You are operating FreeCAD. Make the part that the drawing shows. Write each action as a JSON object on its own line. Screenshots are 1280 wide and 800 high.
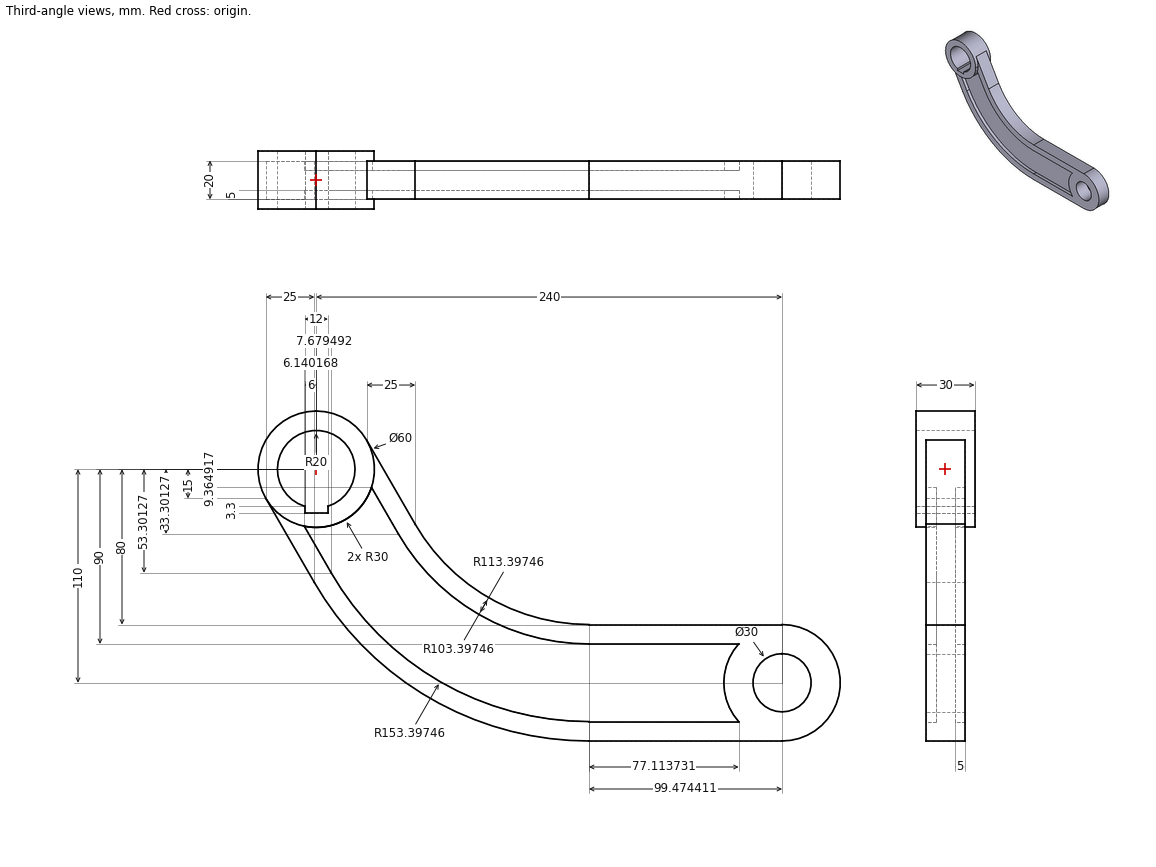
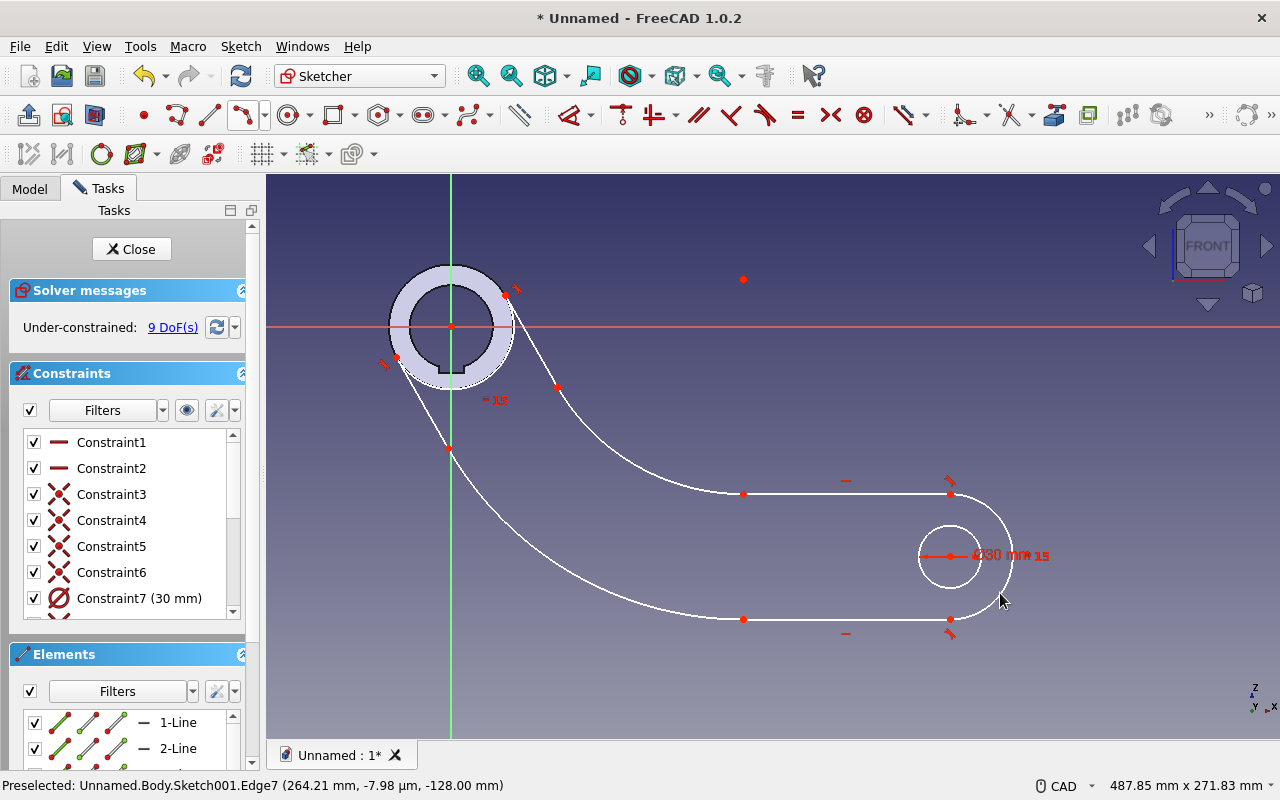
{"action": "left_click", "coordinate": [568, 116]}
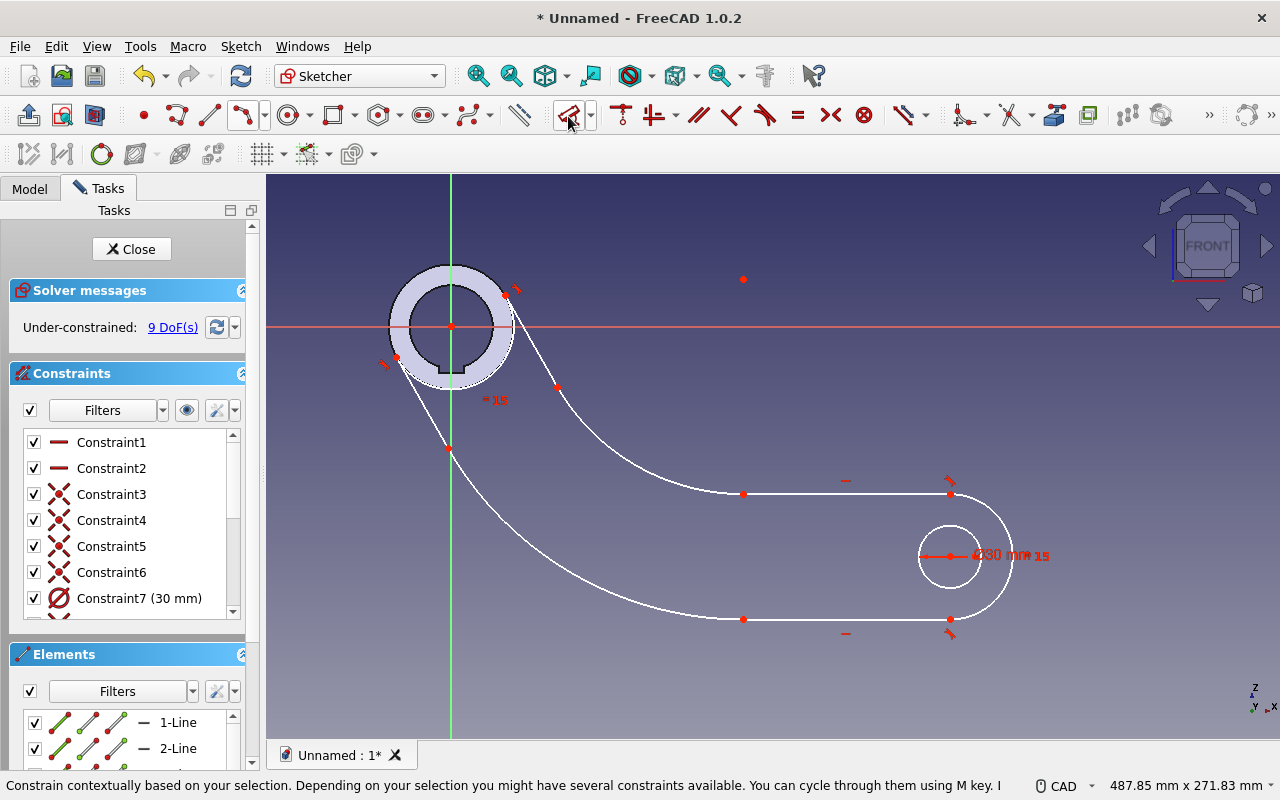
{"action": "left_click", "coordinate": [508, 353]}
{"action": "left_click", "coordinate": [508, 403]}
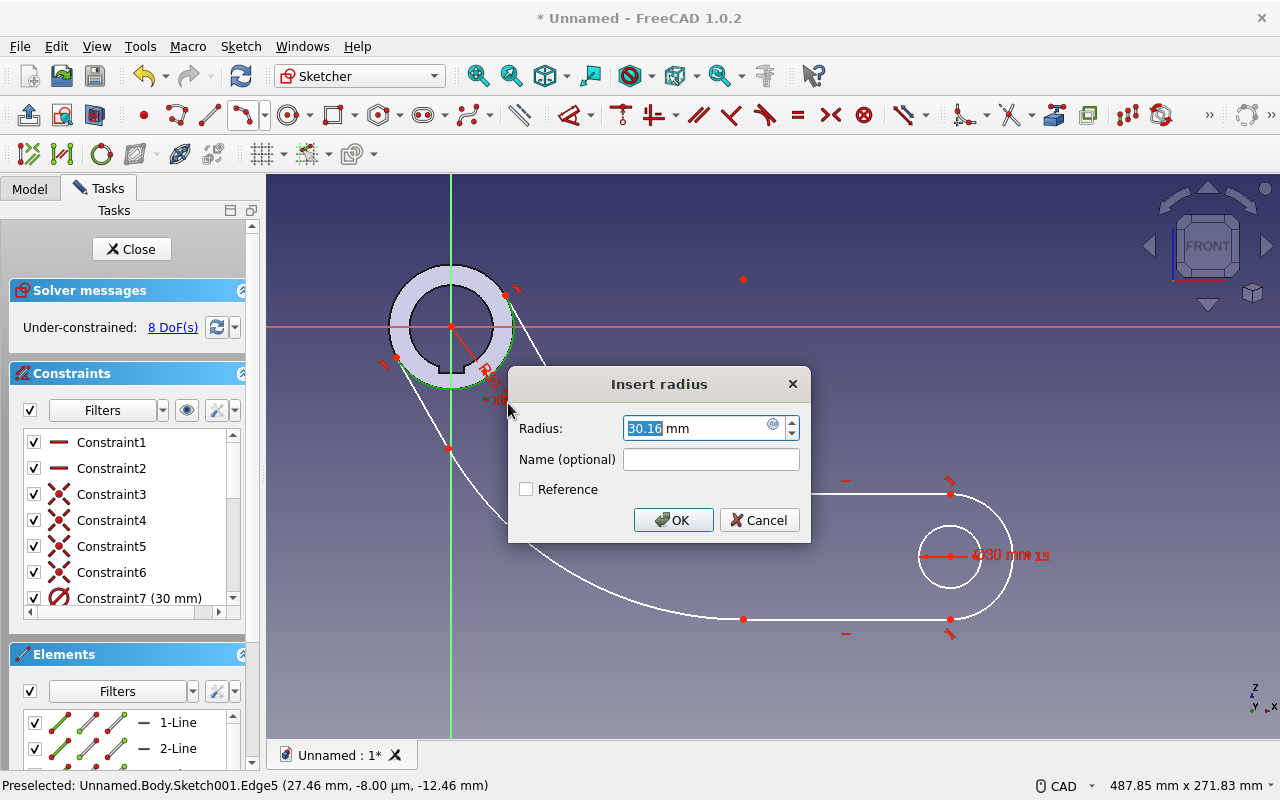
{"action": "type", "text": "30"}
{"action": "key", "text": "Return"}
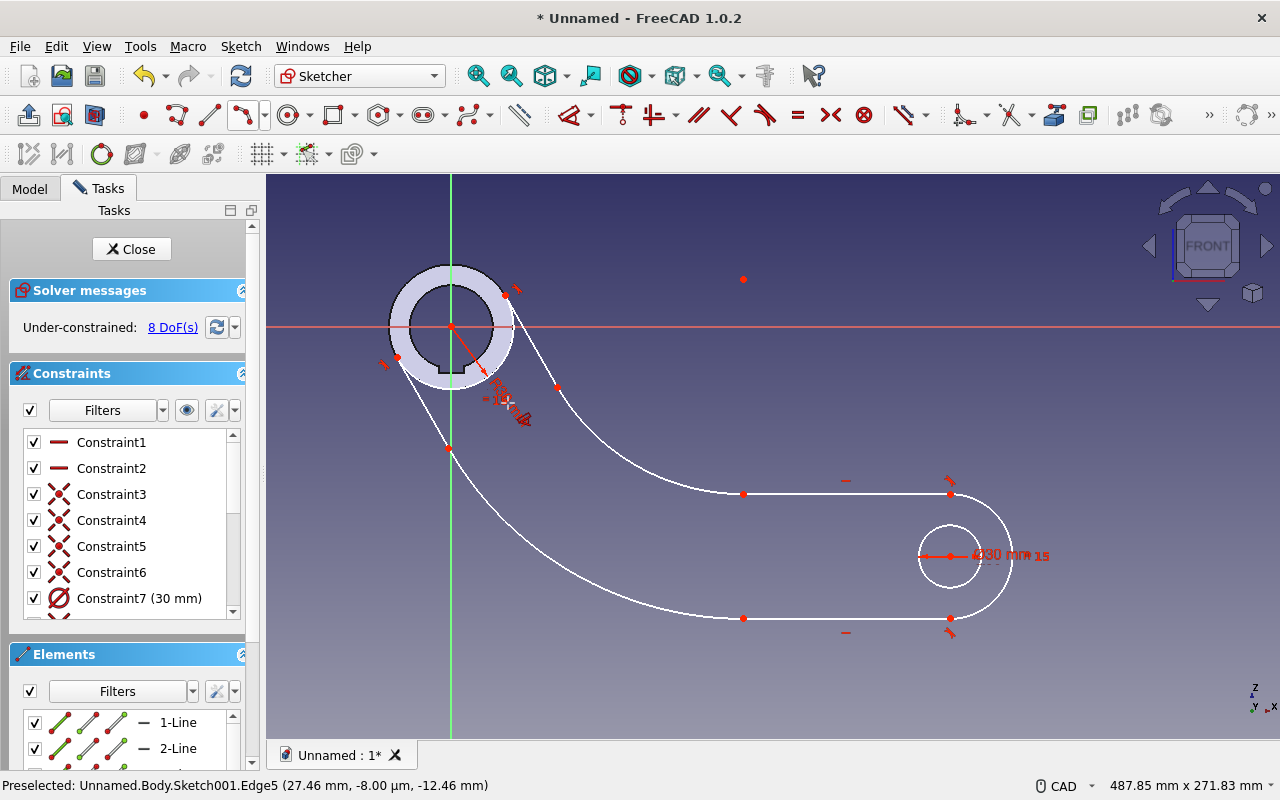
{"action": "left_click", "coordinate": [600, 439]}
{"action": "left_click", "coordinate": [579, 463]}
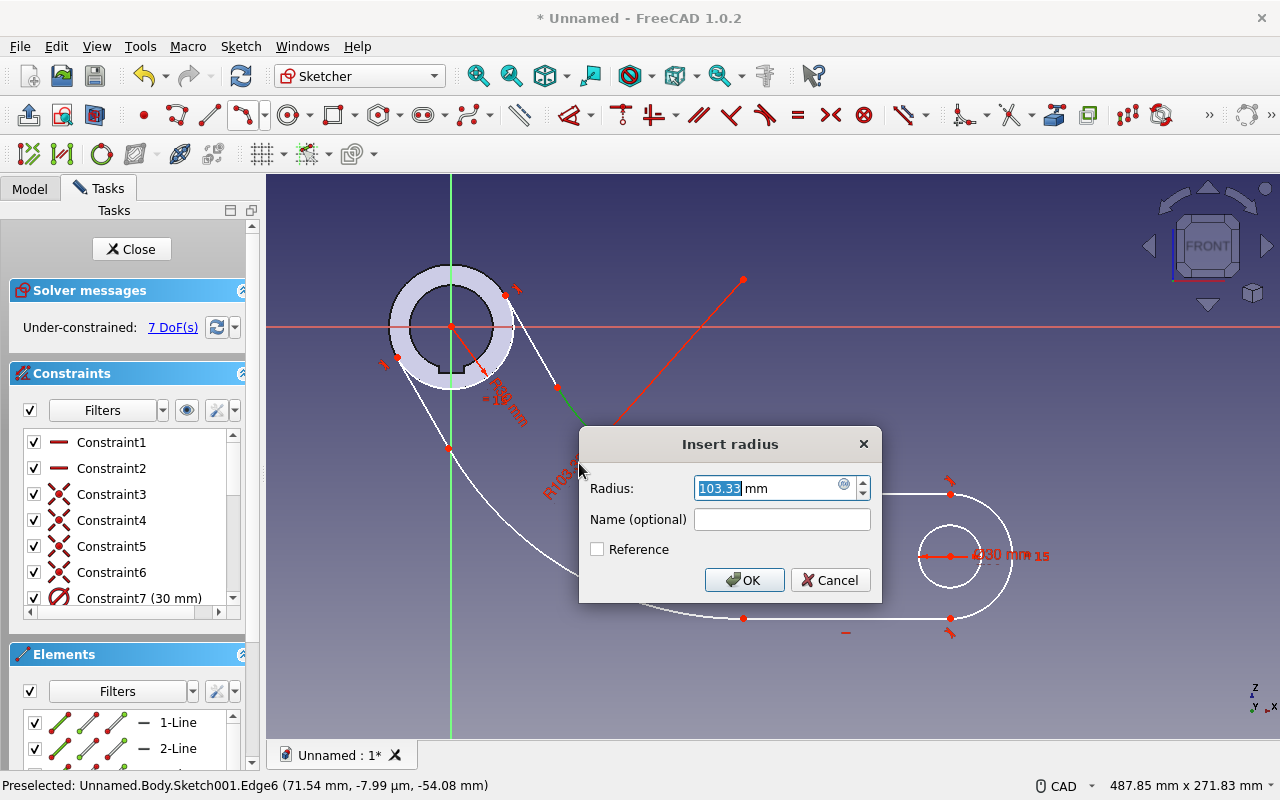
{"action": "type", "text": "103.39746"}
{"action": "key", "text": "Return"}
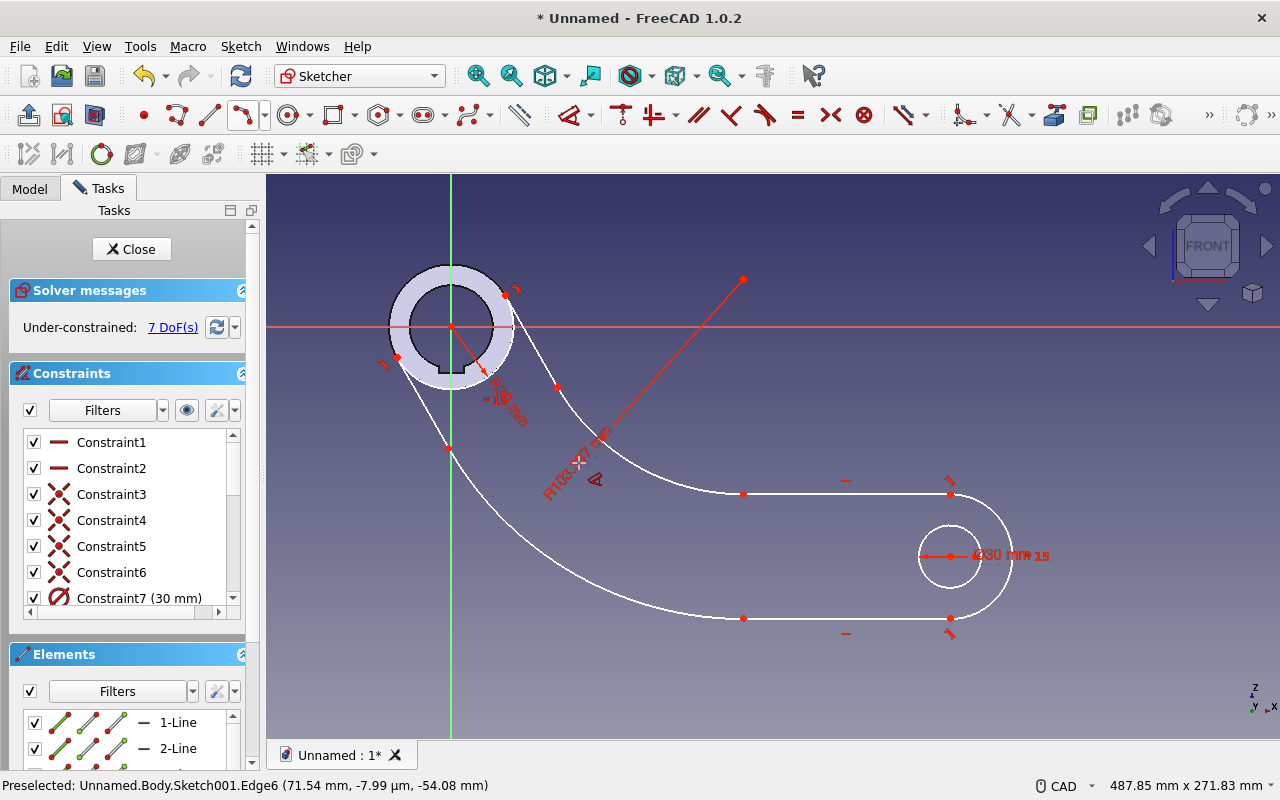
{"action": "scroll", "coordinate": [397, 358], "scroll_direction": "up", "scroll_amount": 2}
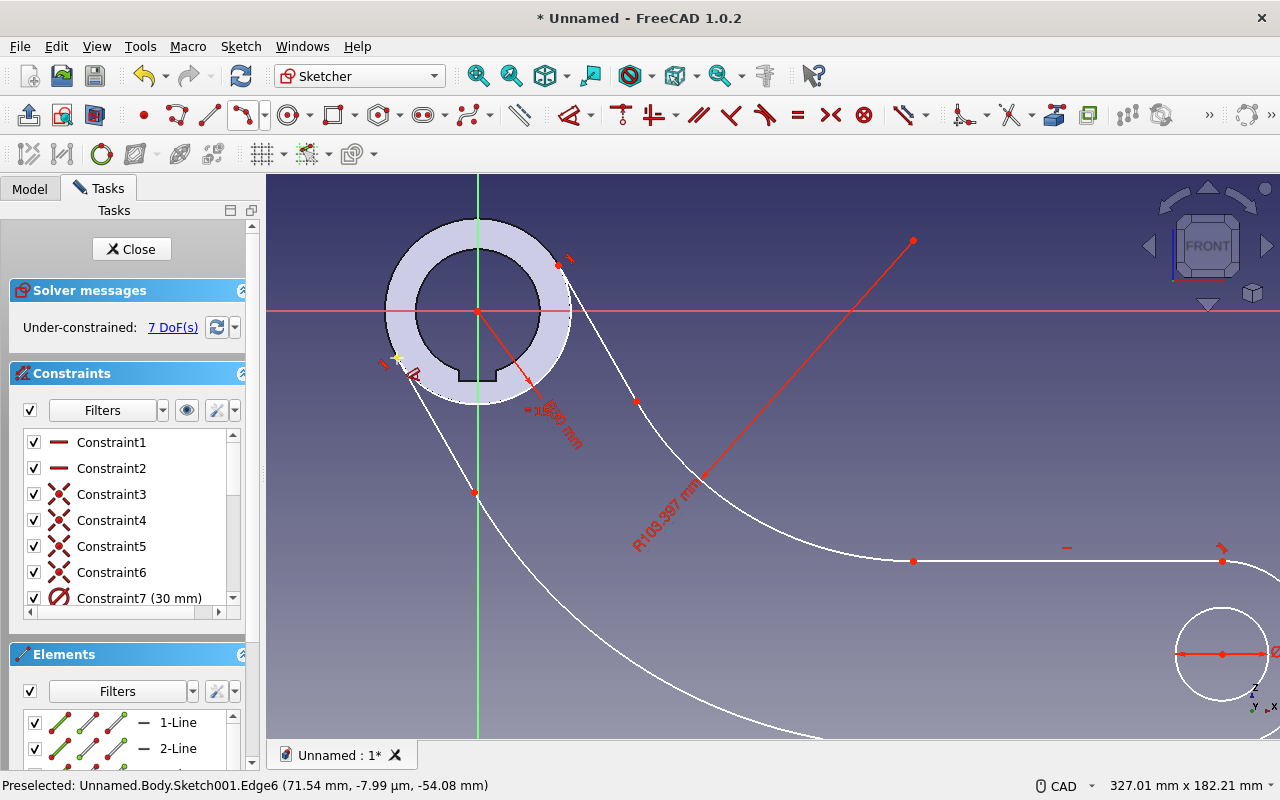
{"action": "left_click", "coordinate": [397, 358]}
{"action": "left_click", "coordinate": [363, 334]}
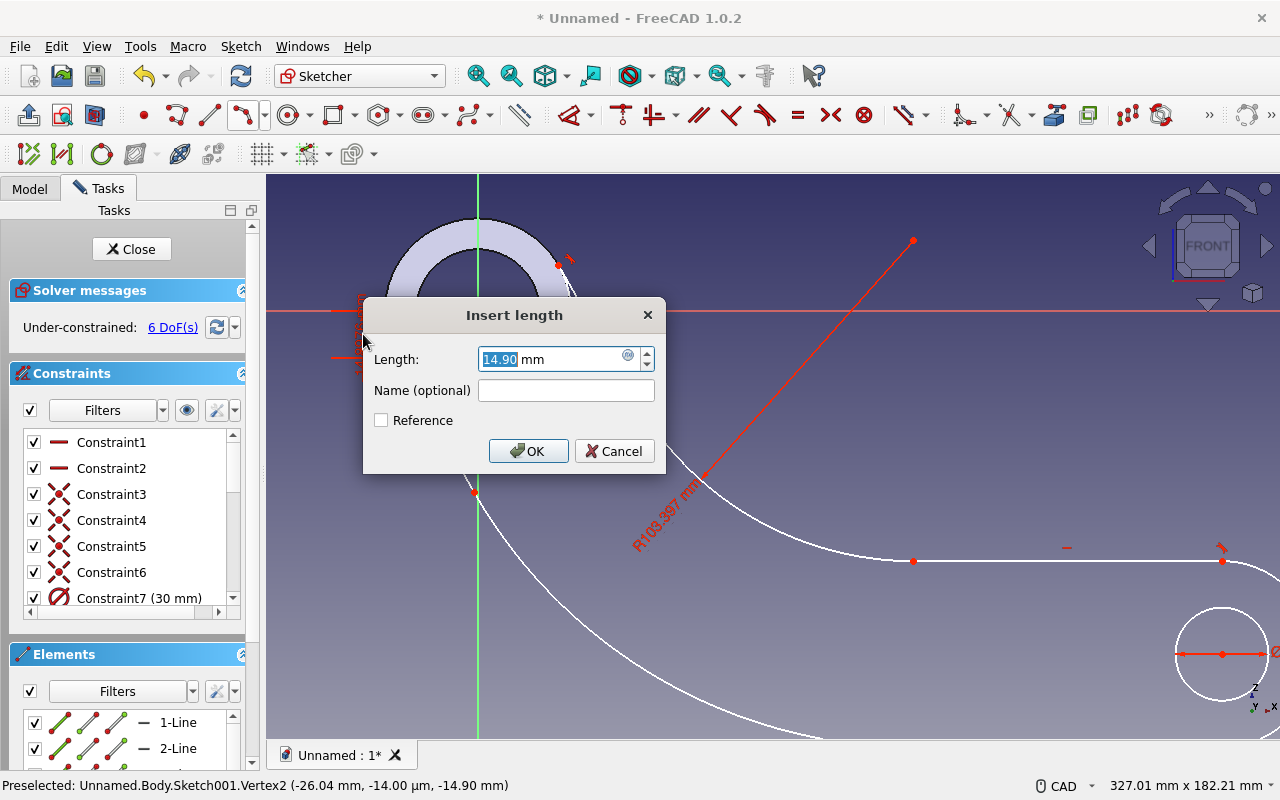
{"action": "type", "text": "15"}
{"action": "key", "text": "Return"}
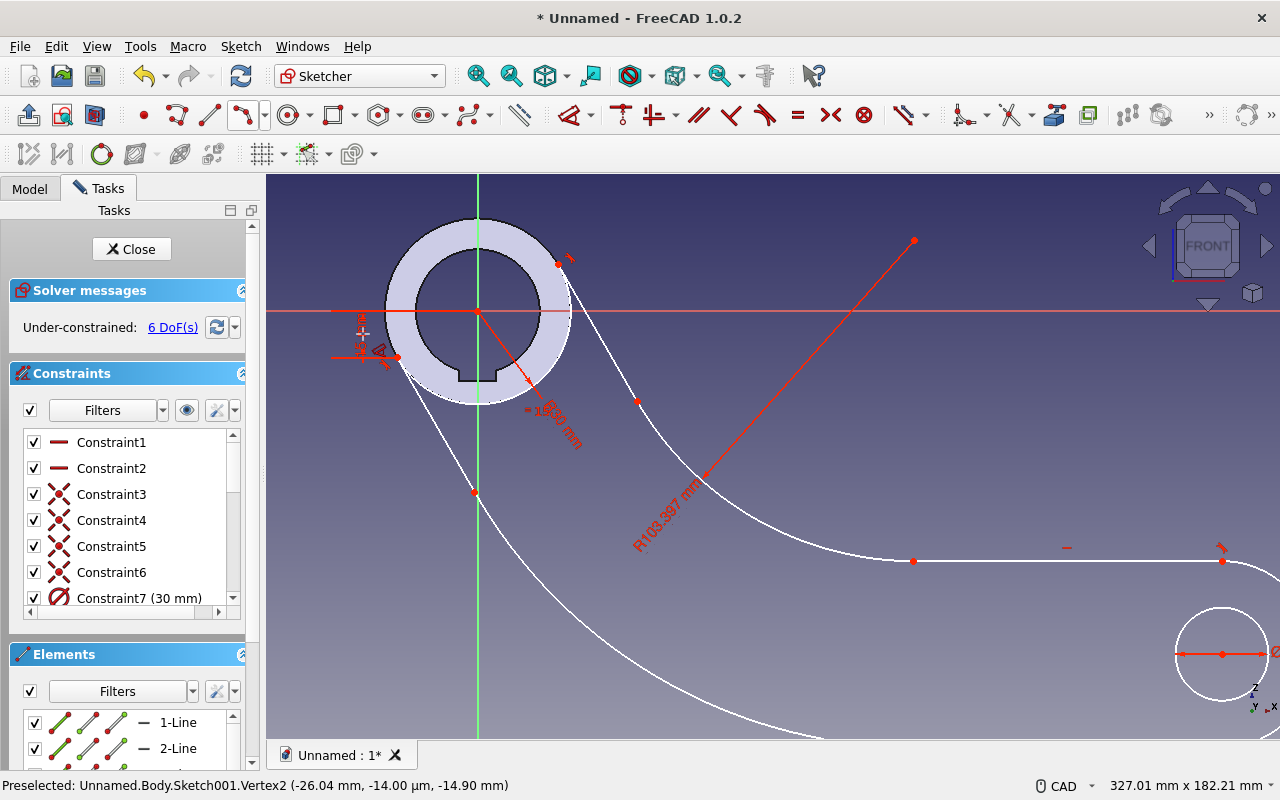
{"action": "left_click", "coordinate": [914, 561]}
{"action": "left_click", "coordinate": [444, 379]}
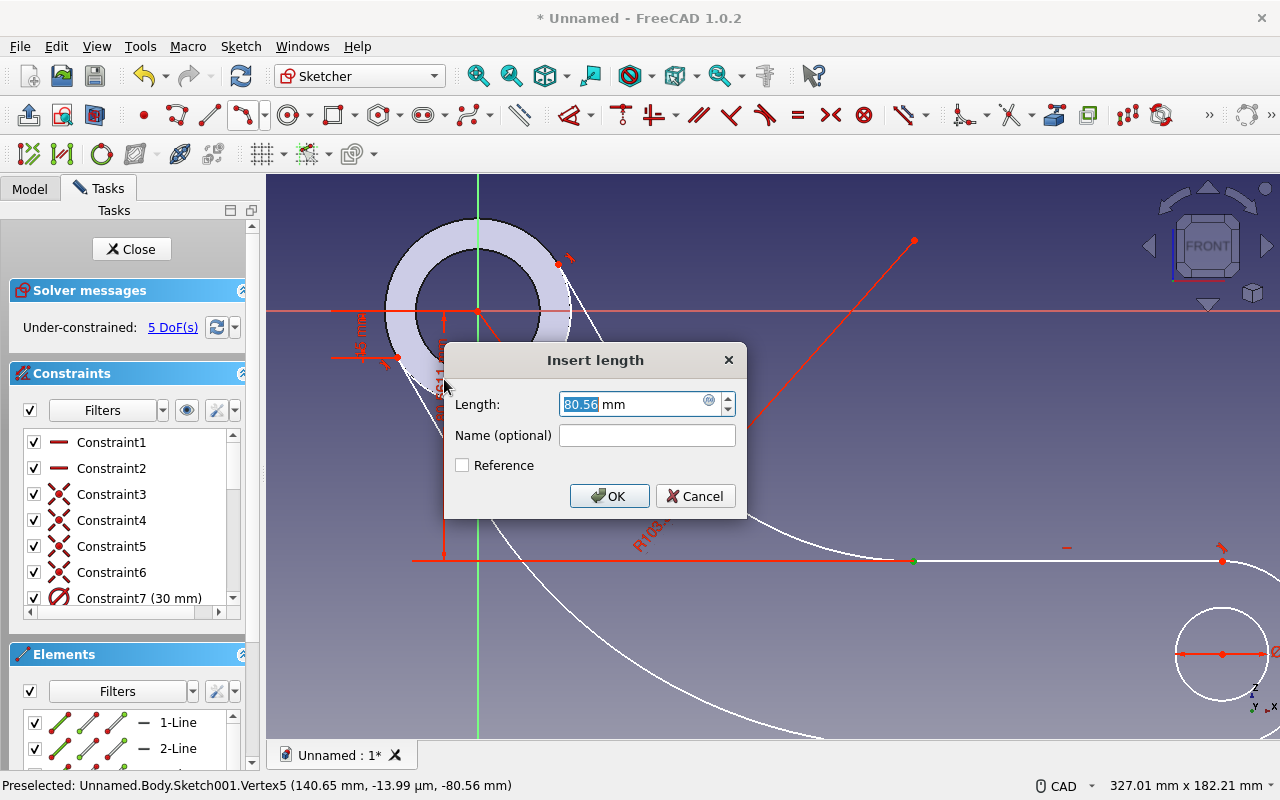
{"action": "type", "text": "80"}
{"action": "key", "text": "Return"}